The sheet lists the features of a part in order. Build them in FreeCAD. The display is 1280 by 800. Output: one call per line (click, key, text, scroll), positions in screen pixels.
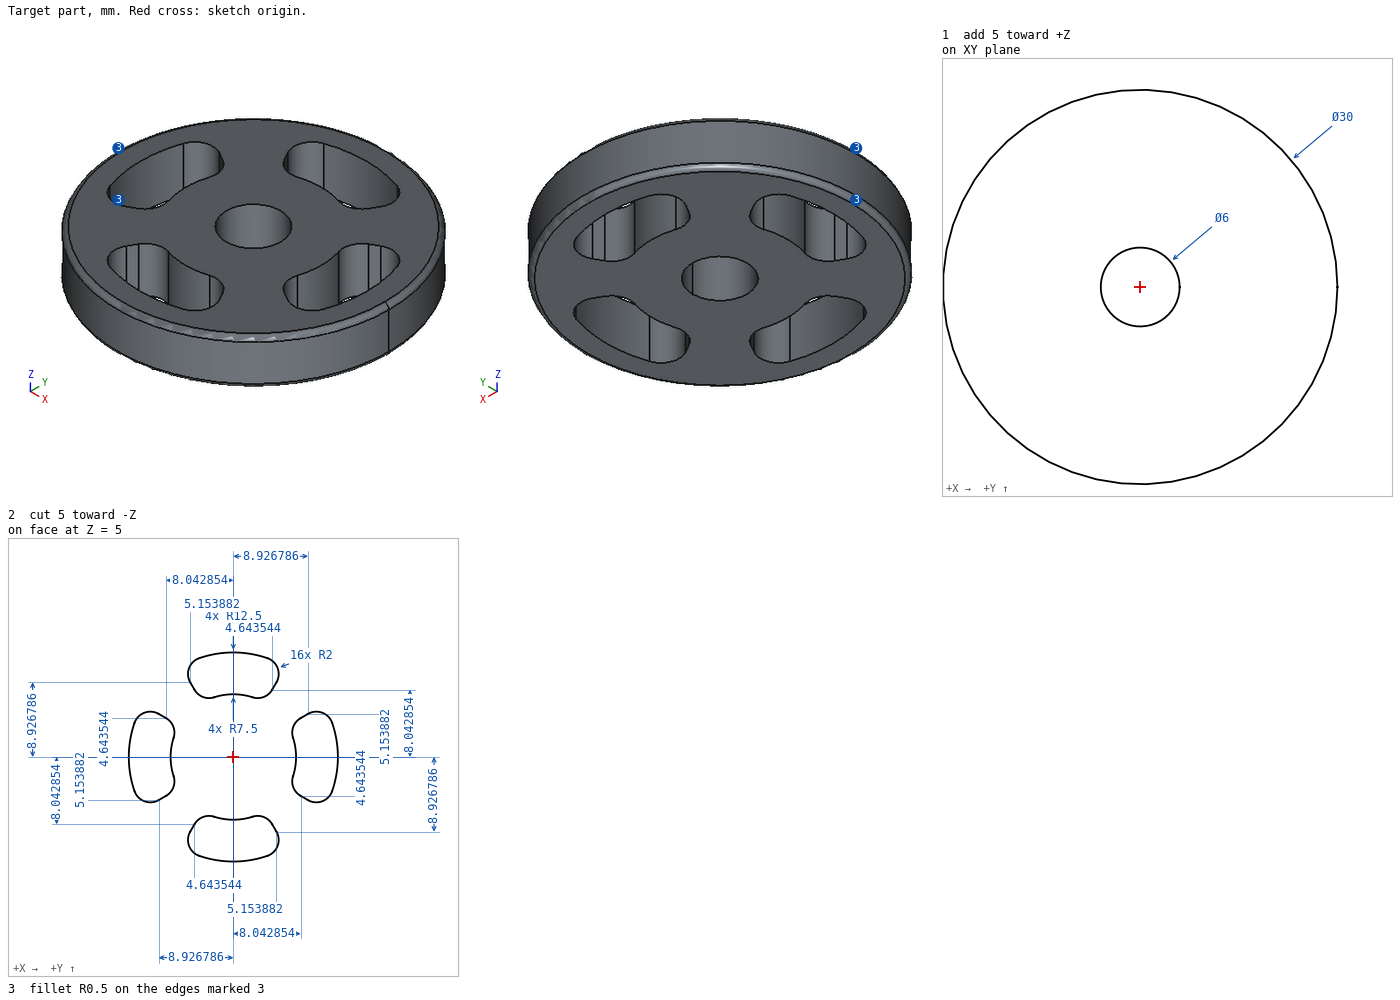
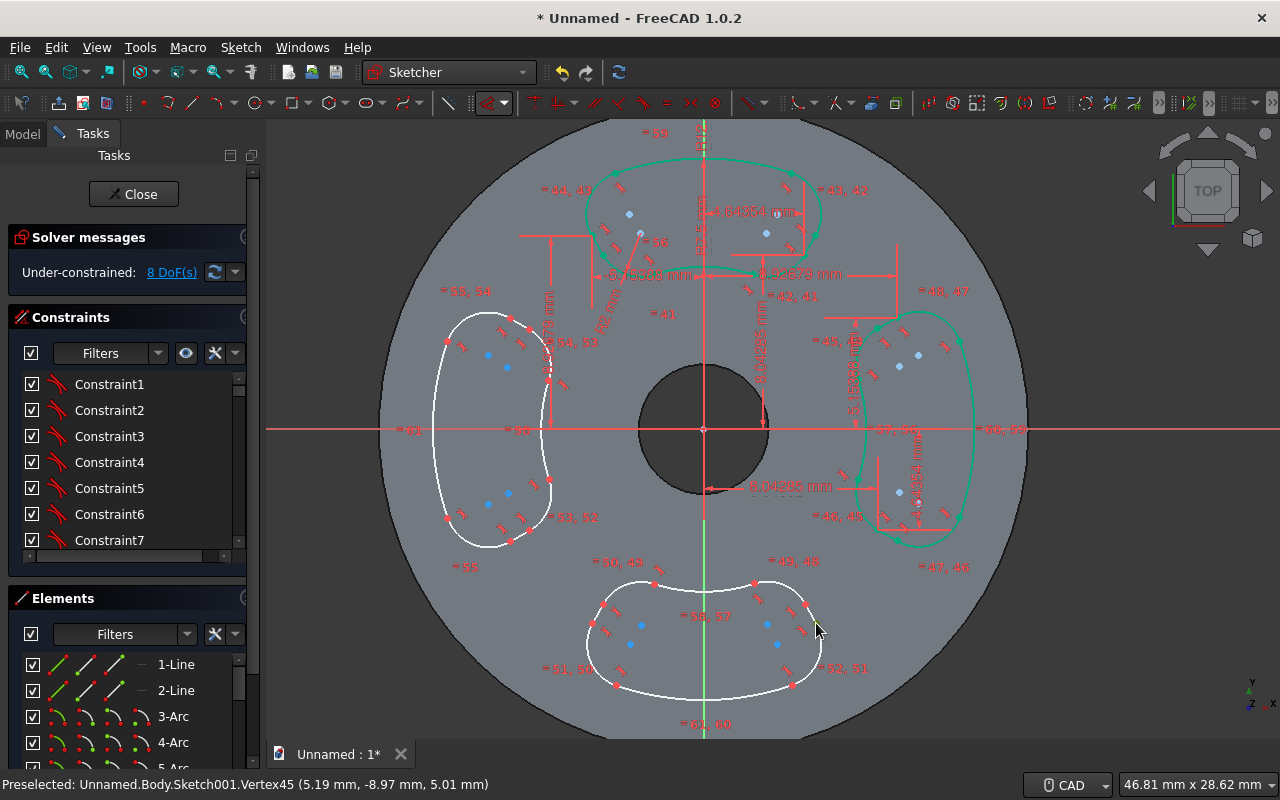
key(l)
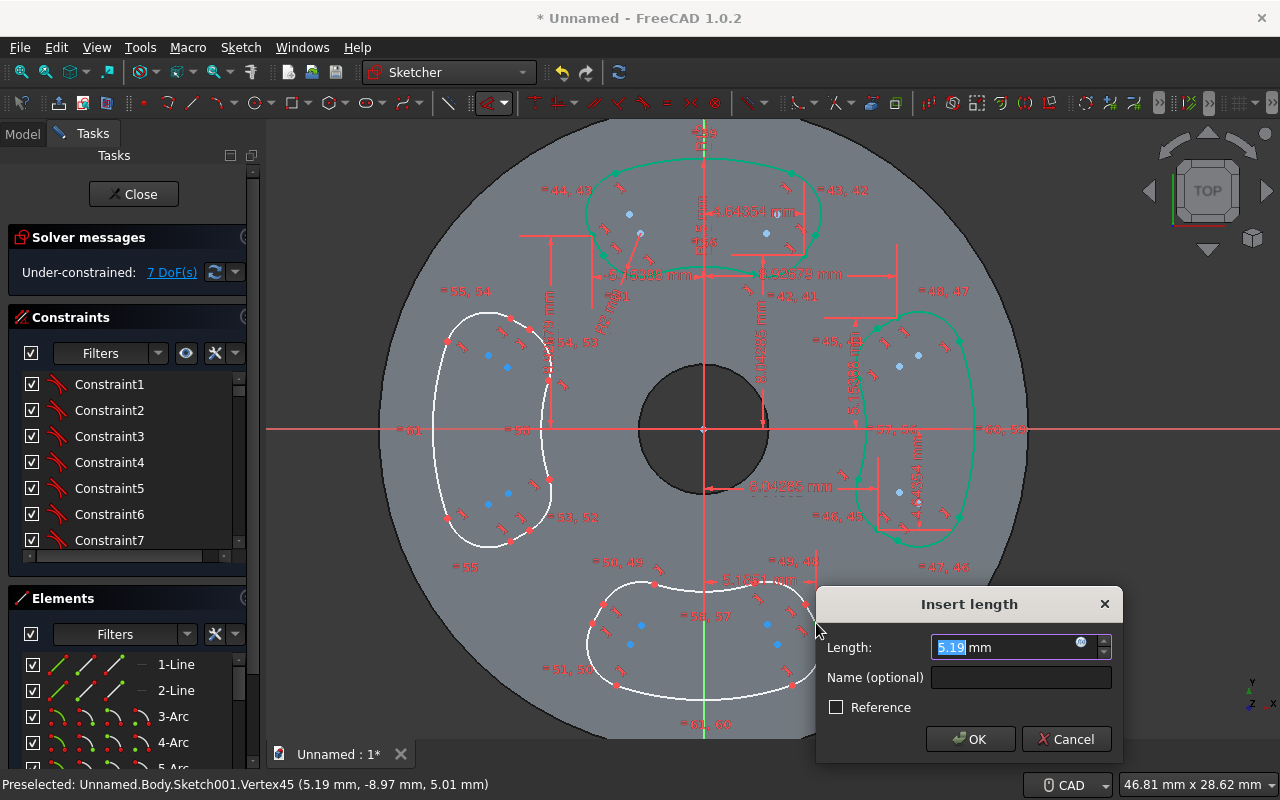
text(5.153882)
key(Return)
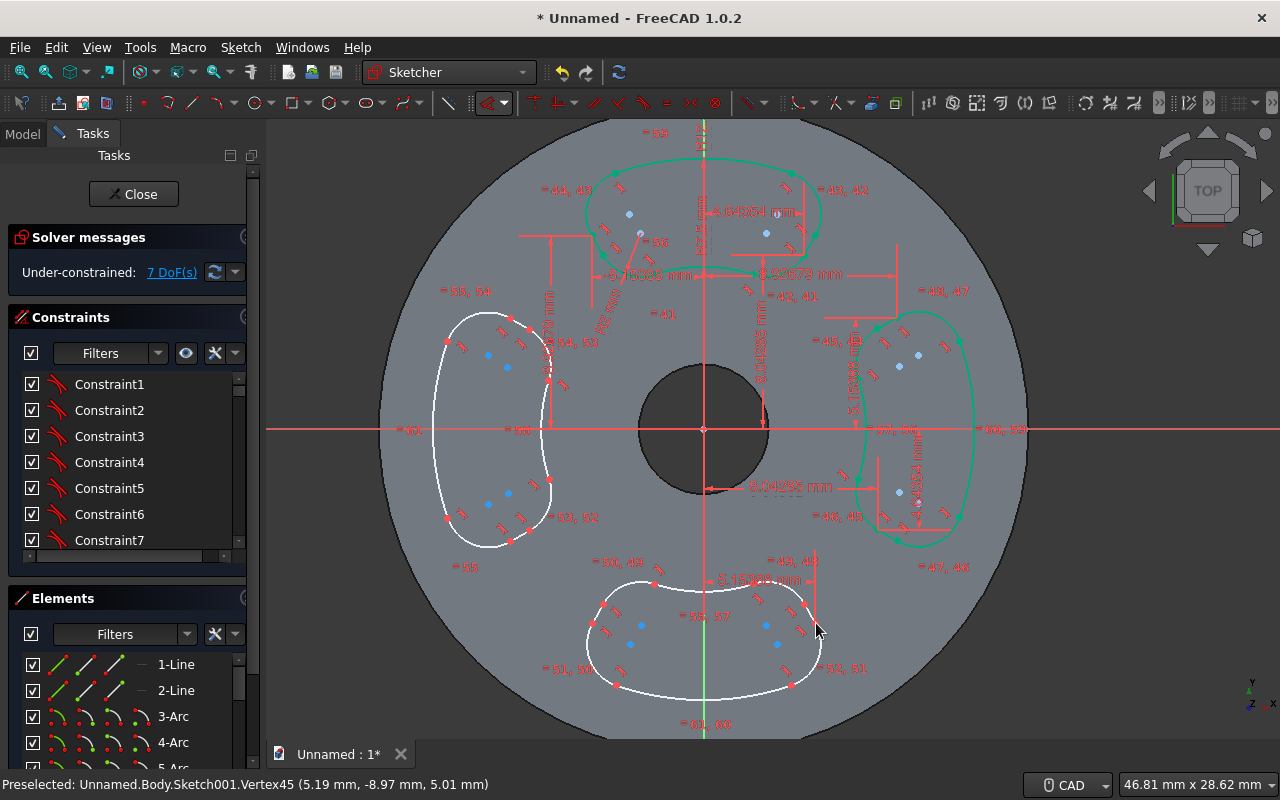
click(815, 623)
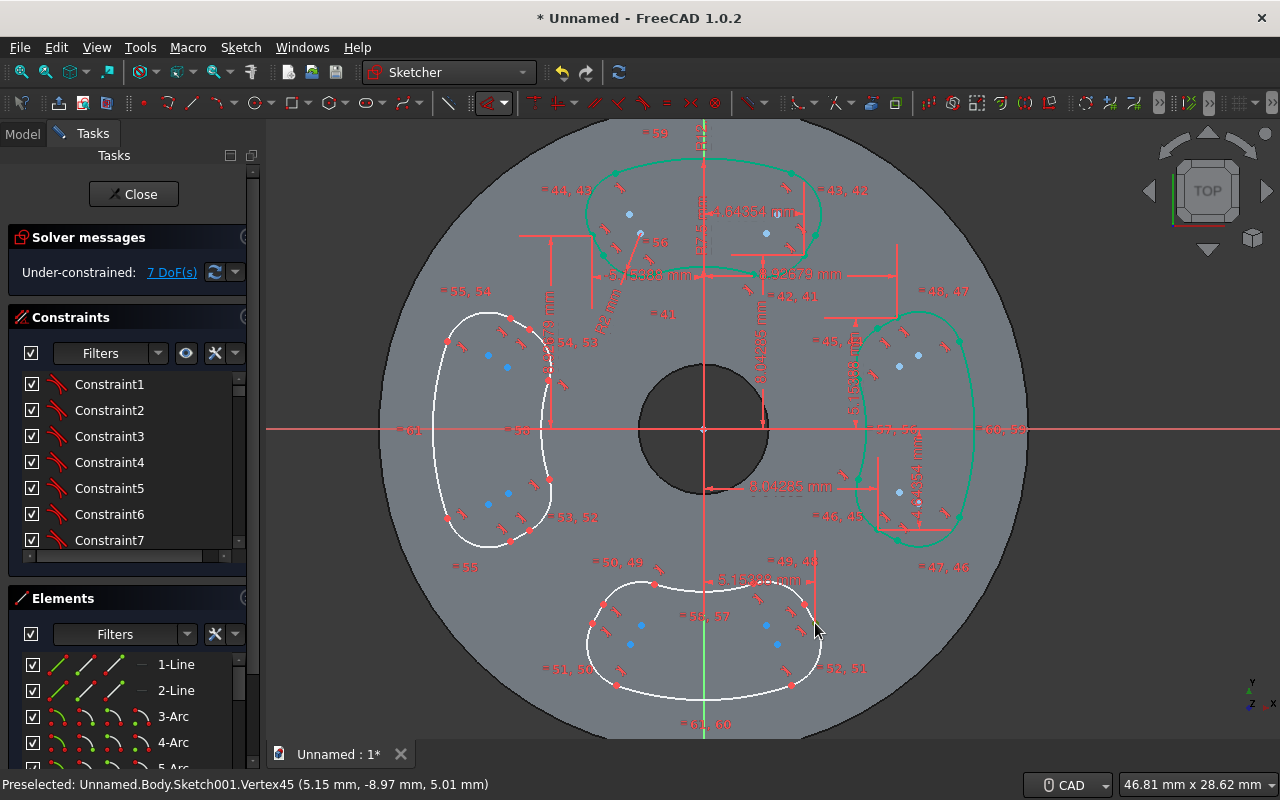
click(506, 104)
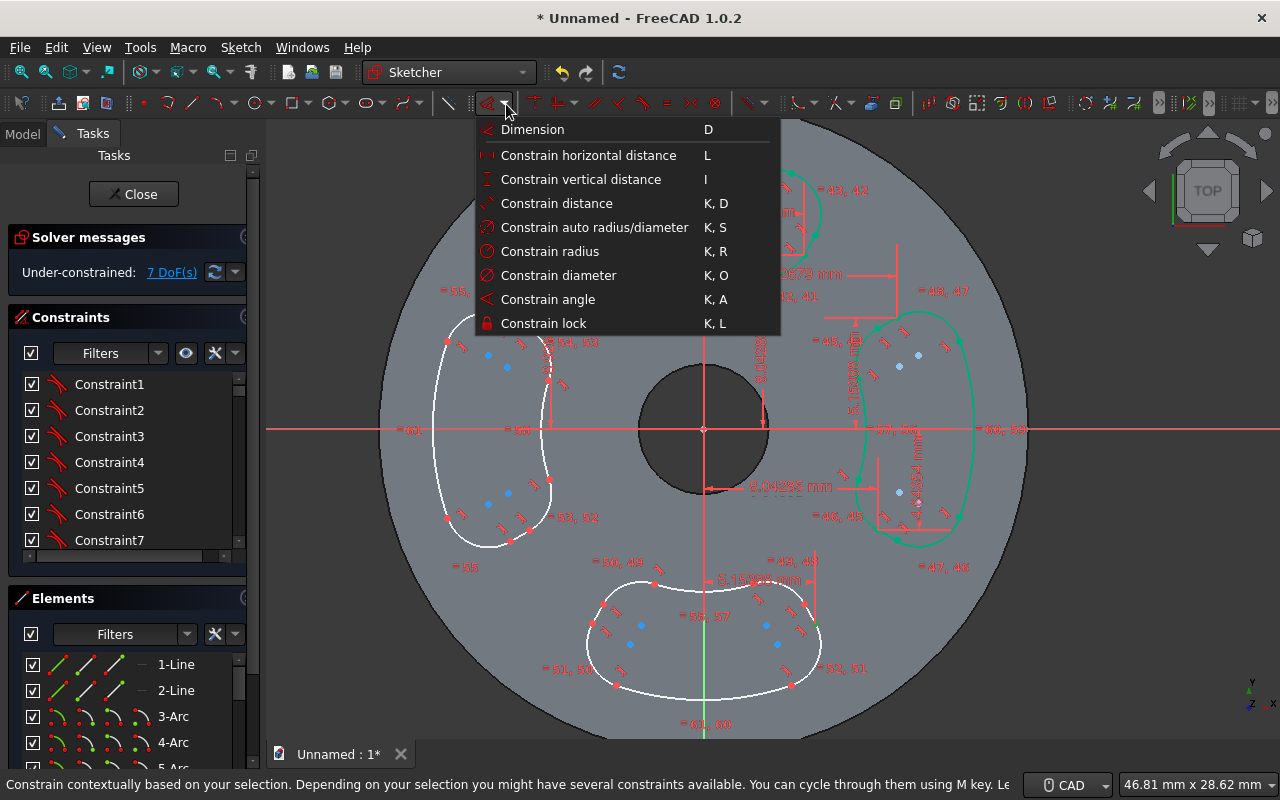
click(628, 179)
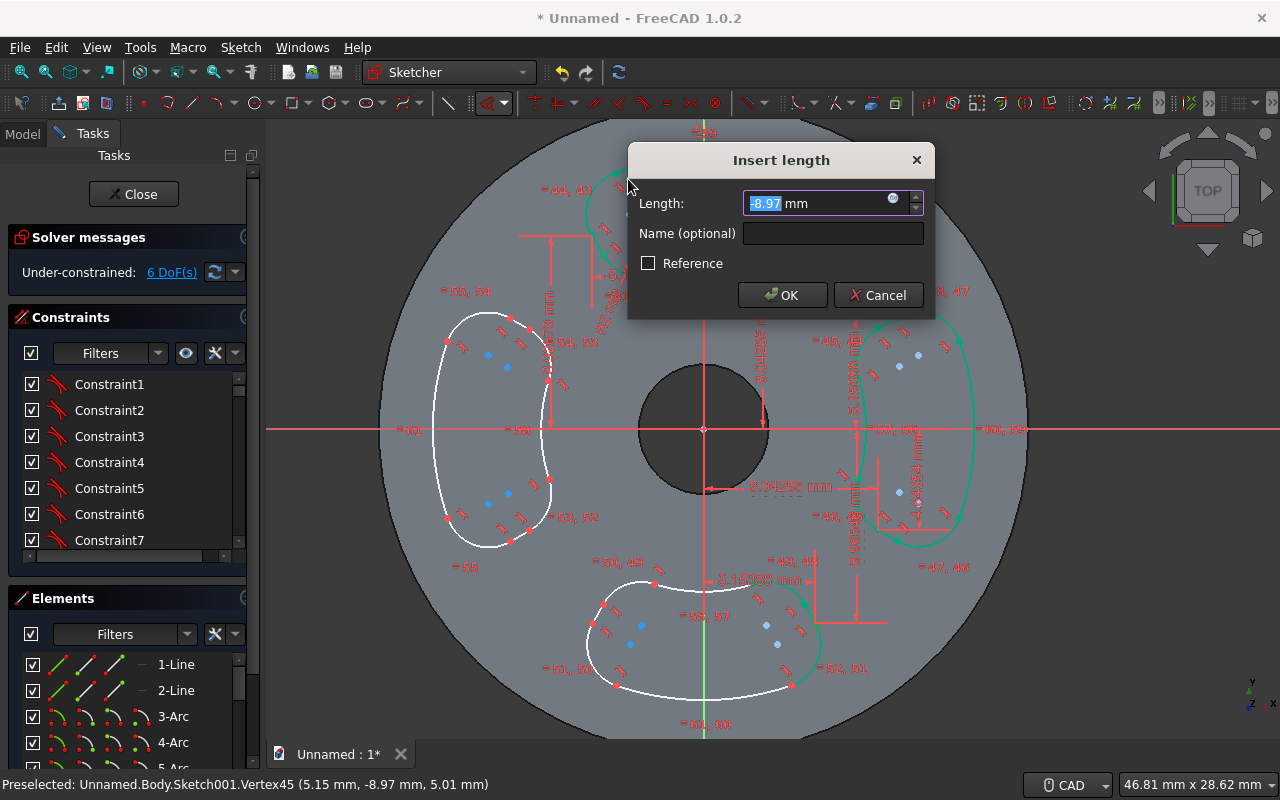
text(-8.926786)
key(Return)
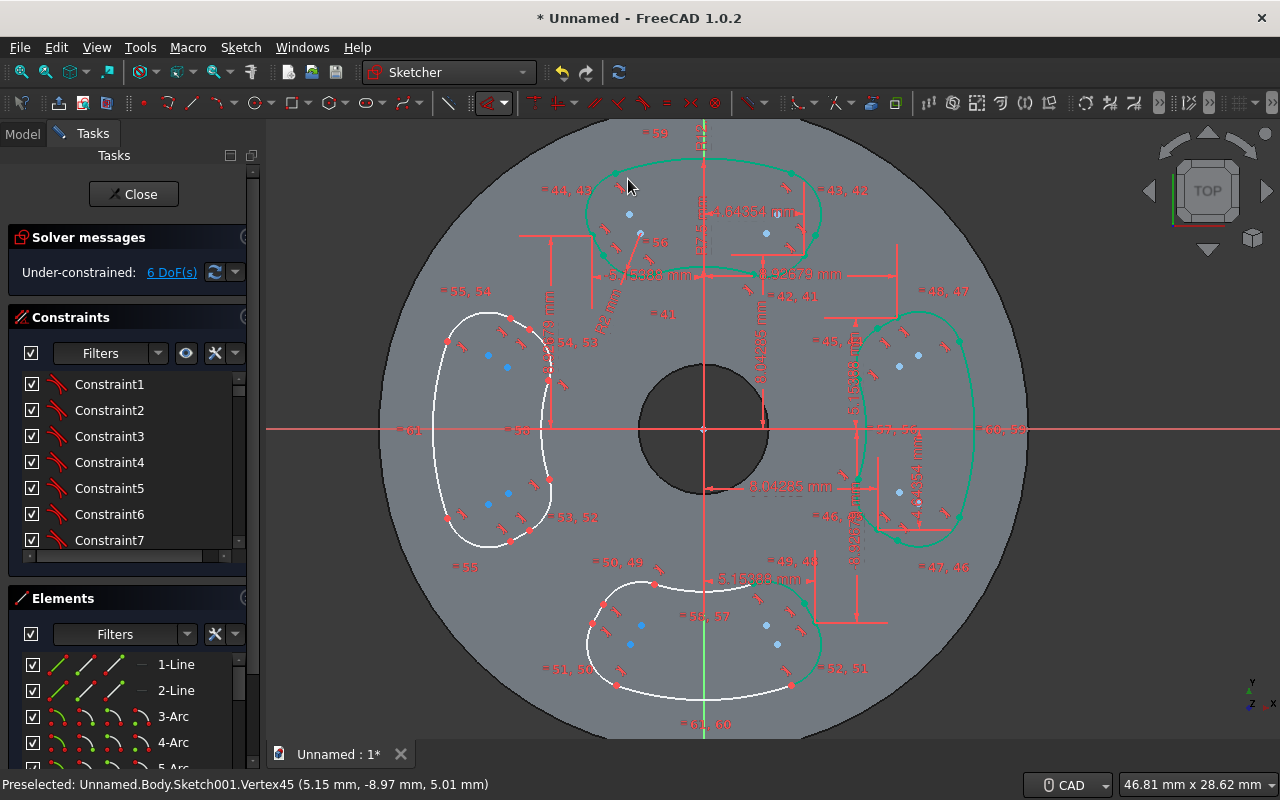
click(603, 604)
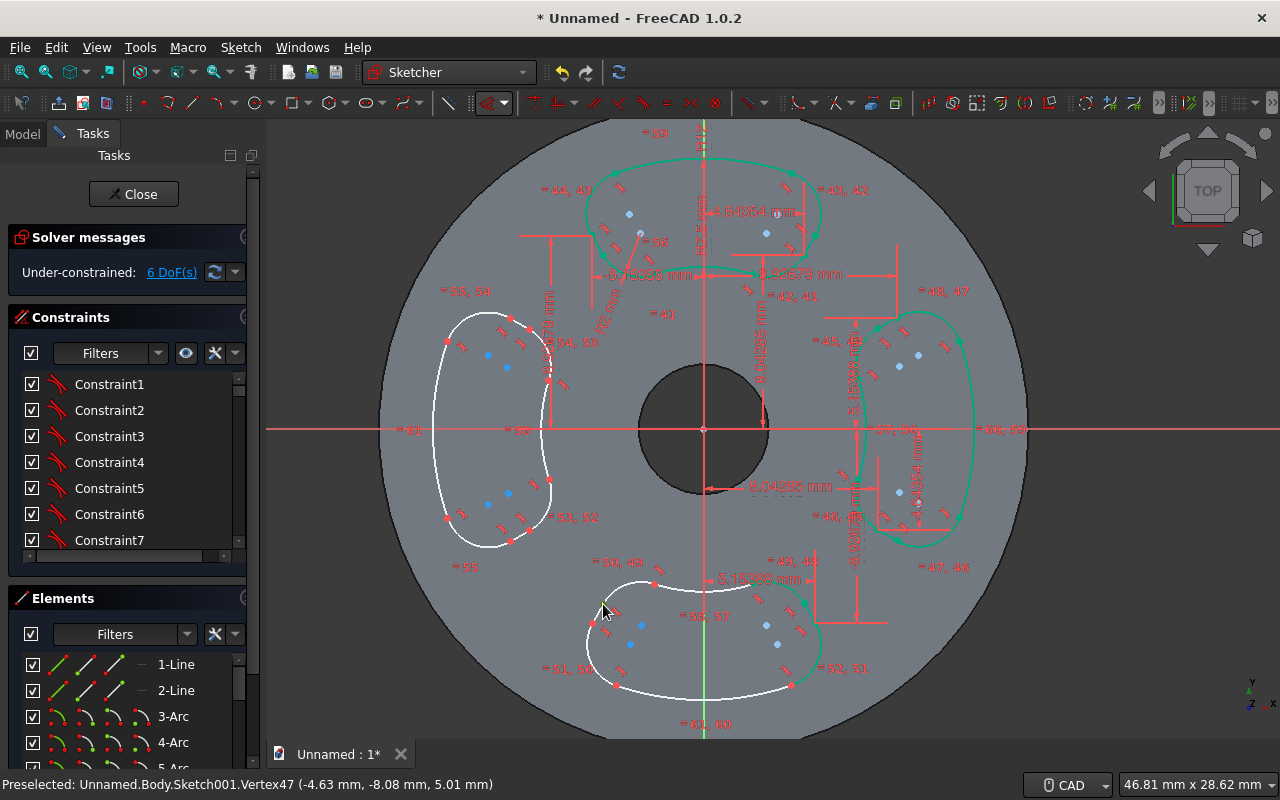
key(l)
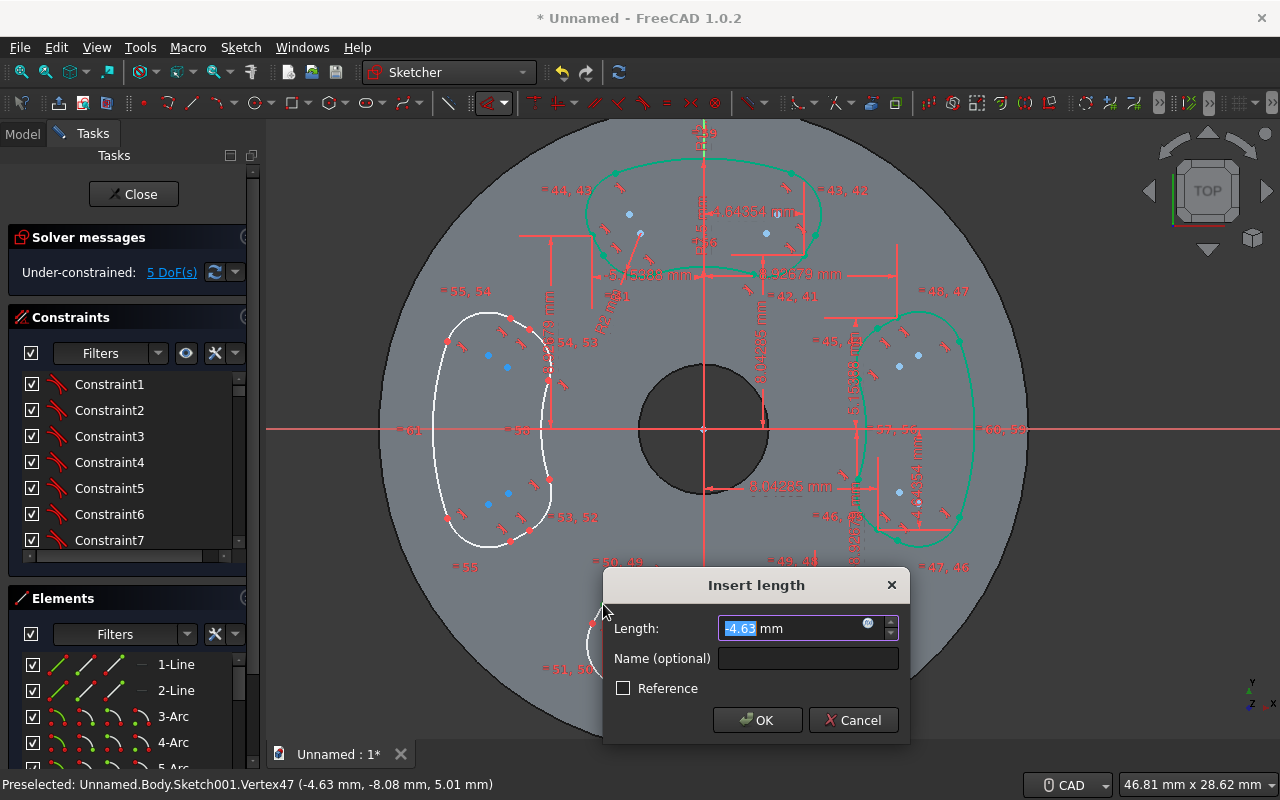
text(-4.643544)
key(Return)